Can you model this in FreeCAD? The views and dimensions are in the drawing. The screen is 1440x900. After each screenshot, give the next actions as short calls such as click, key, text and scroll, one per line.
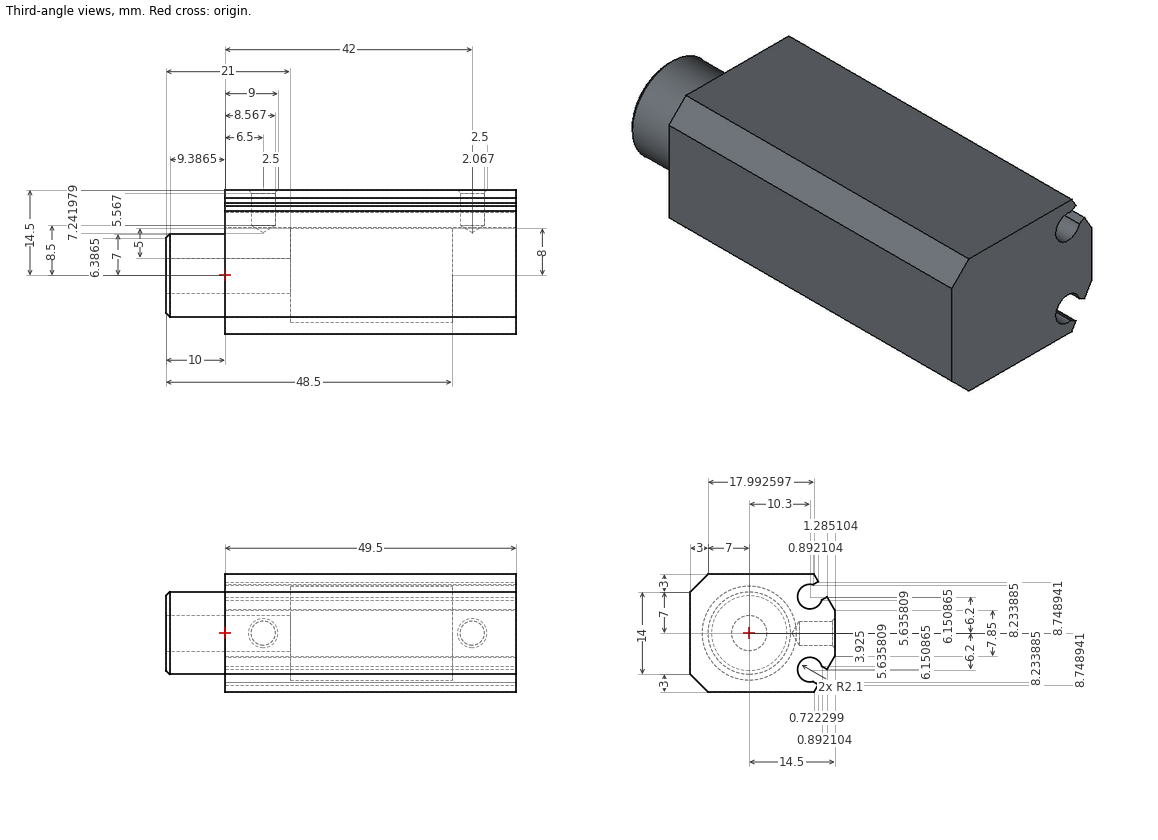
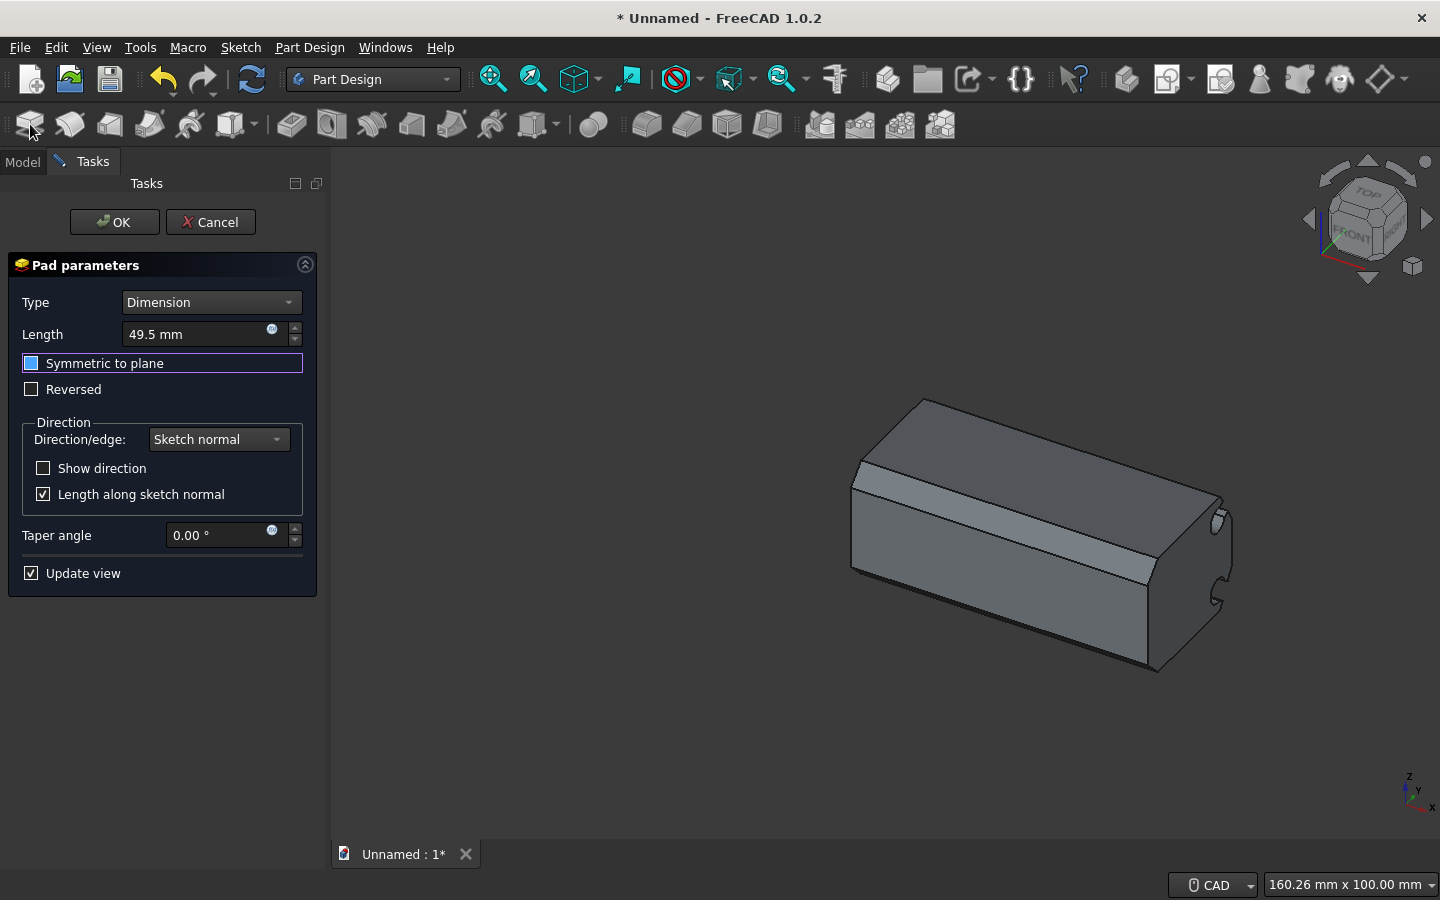
click(115, 222)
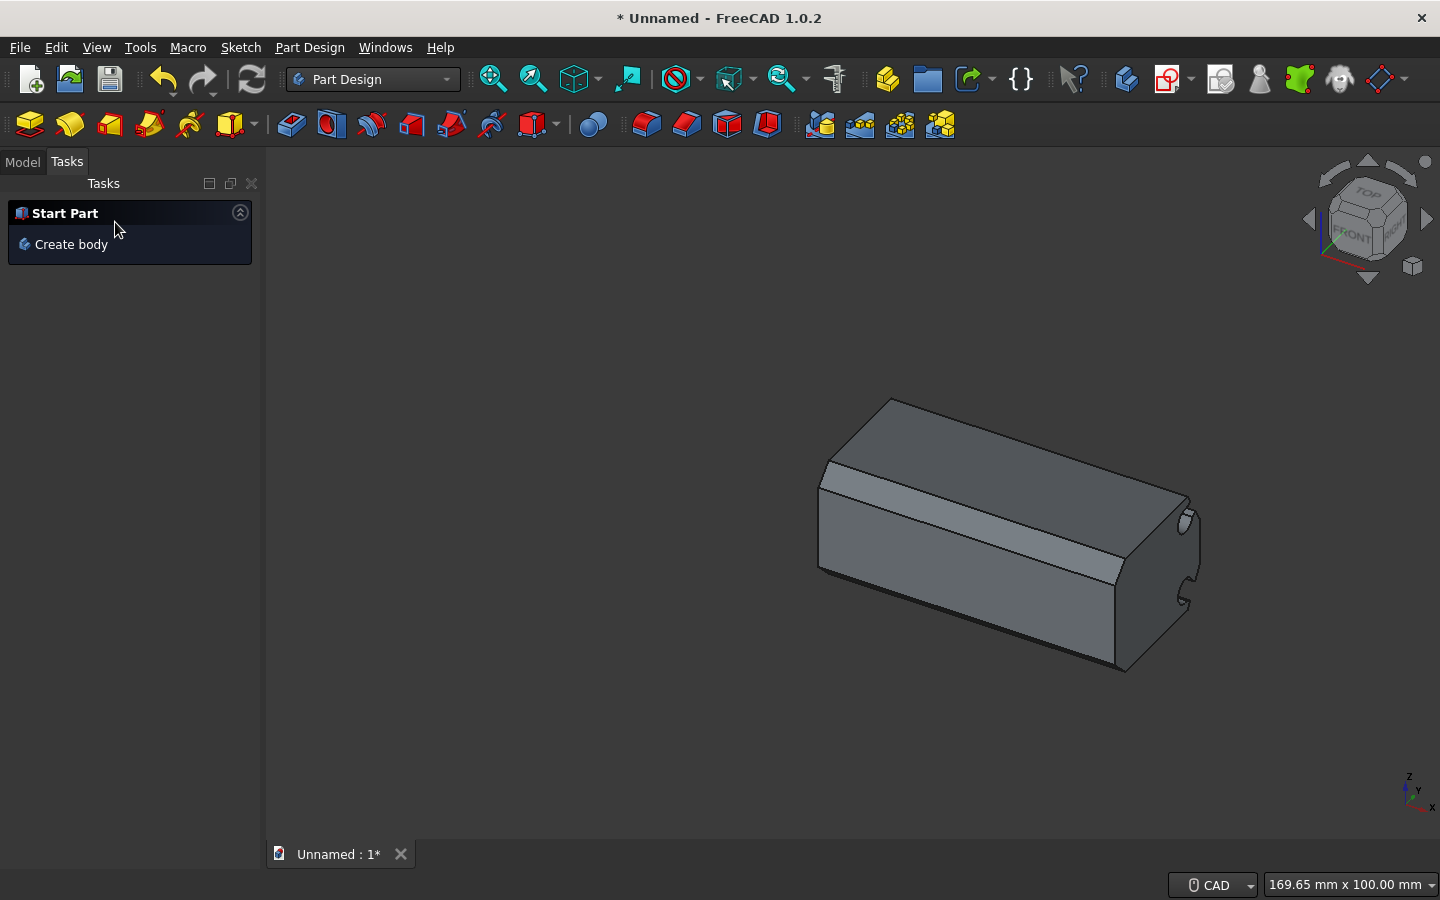
key(v)
key(f)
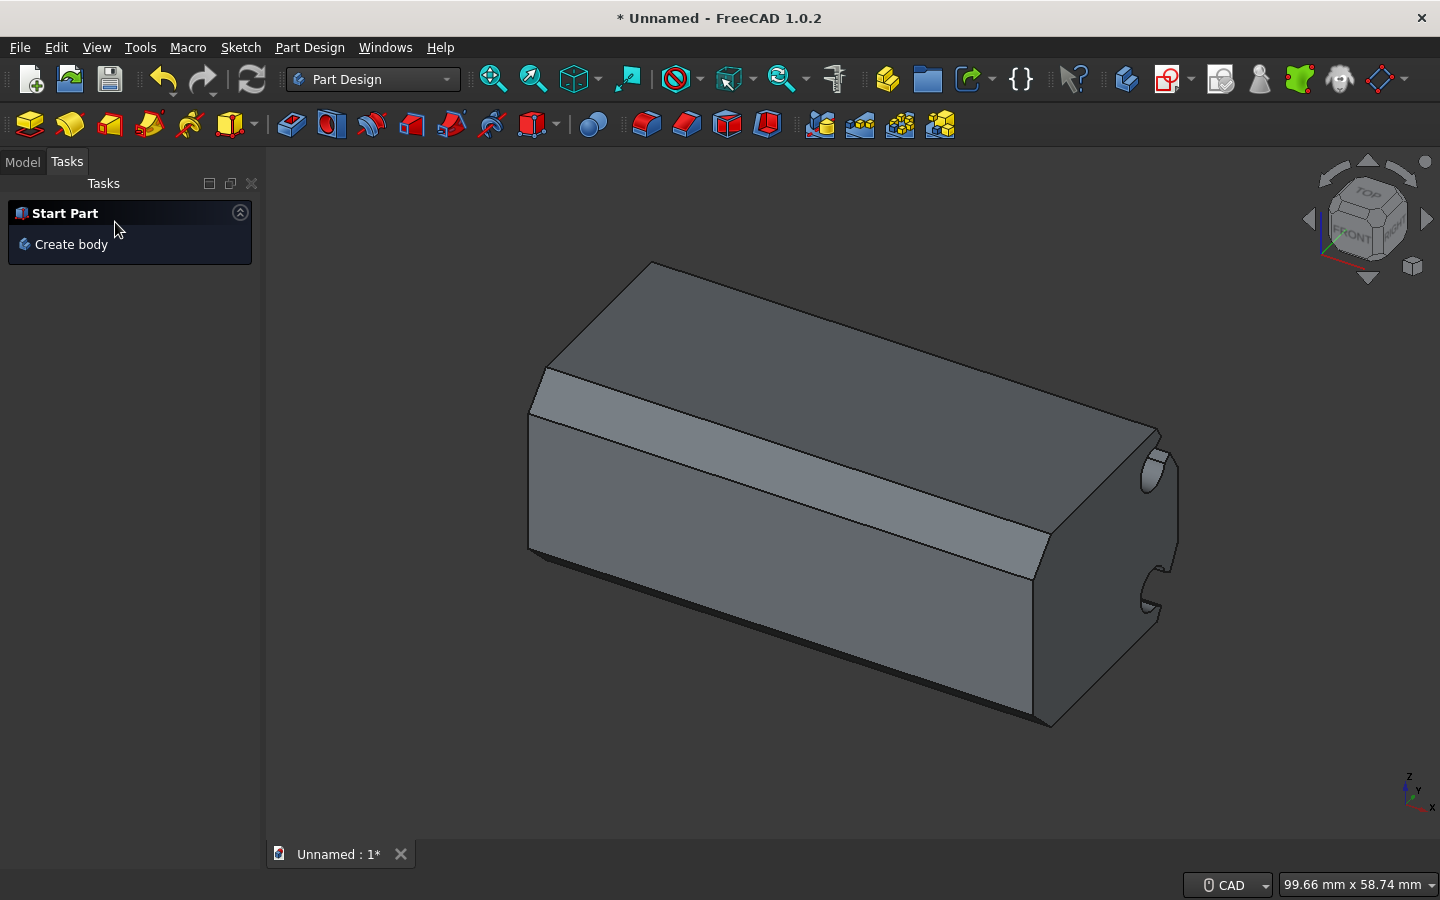
click(1168, 80)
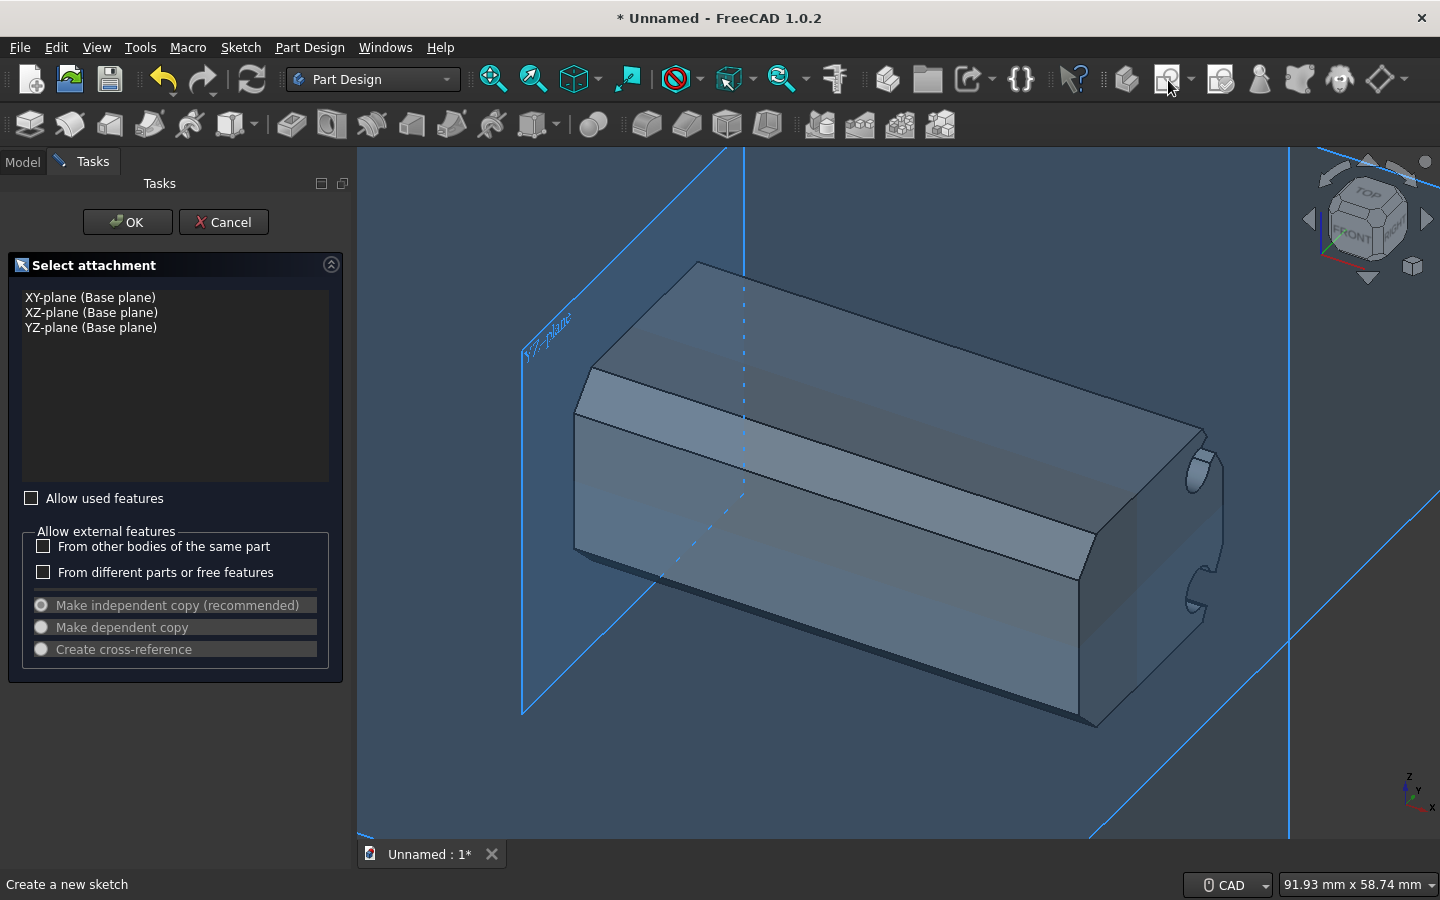
click(82, 298)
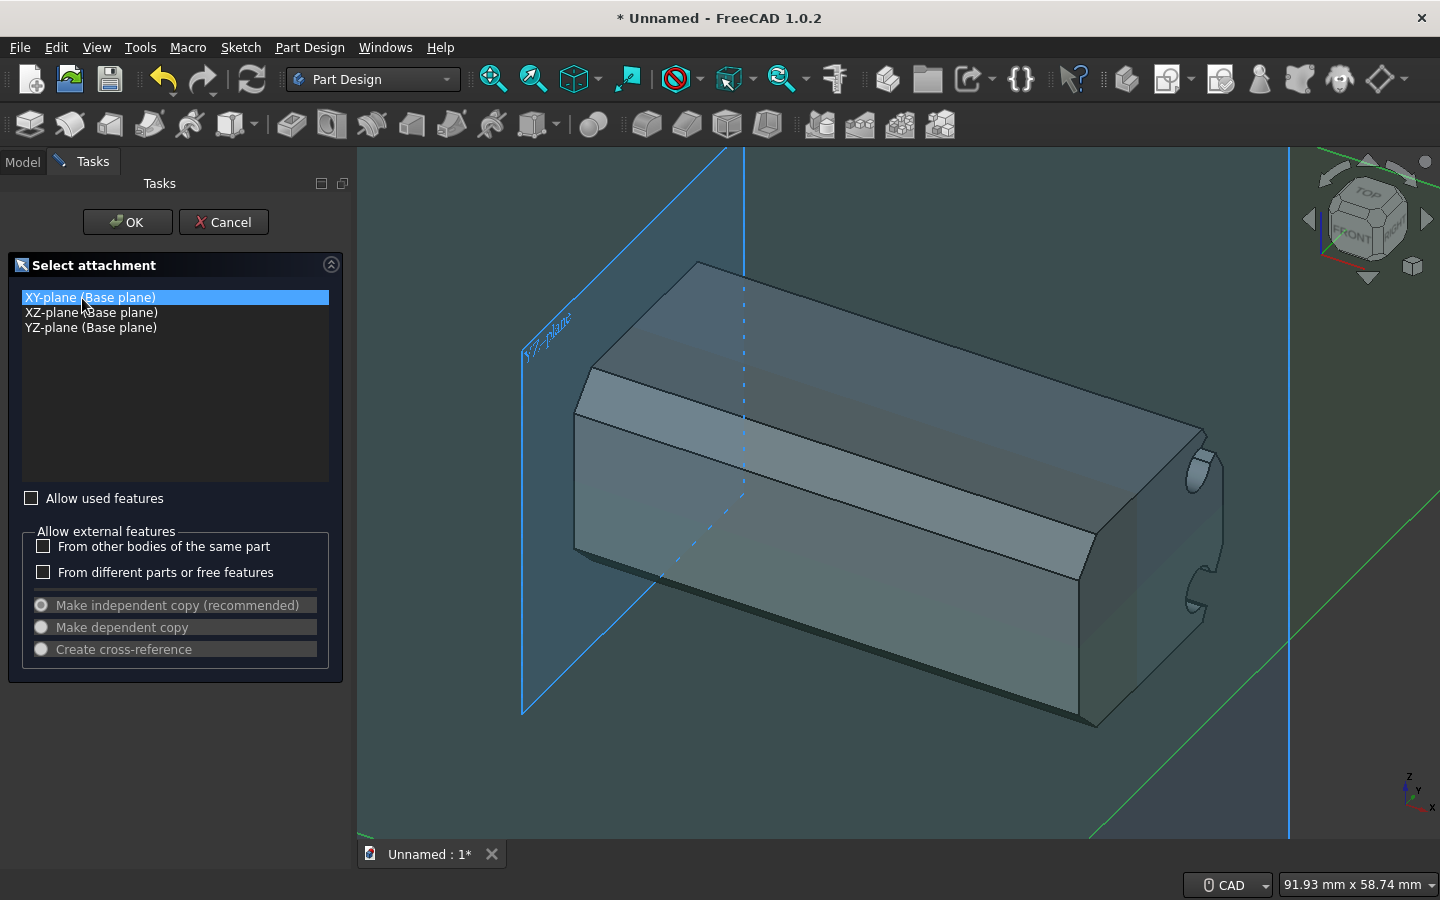
click(128, 222)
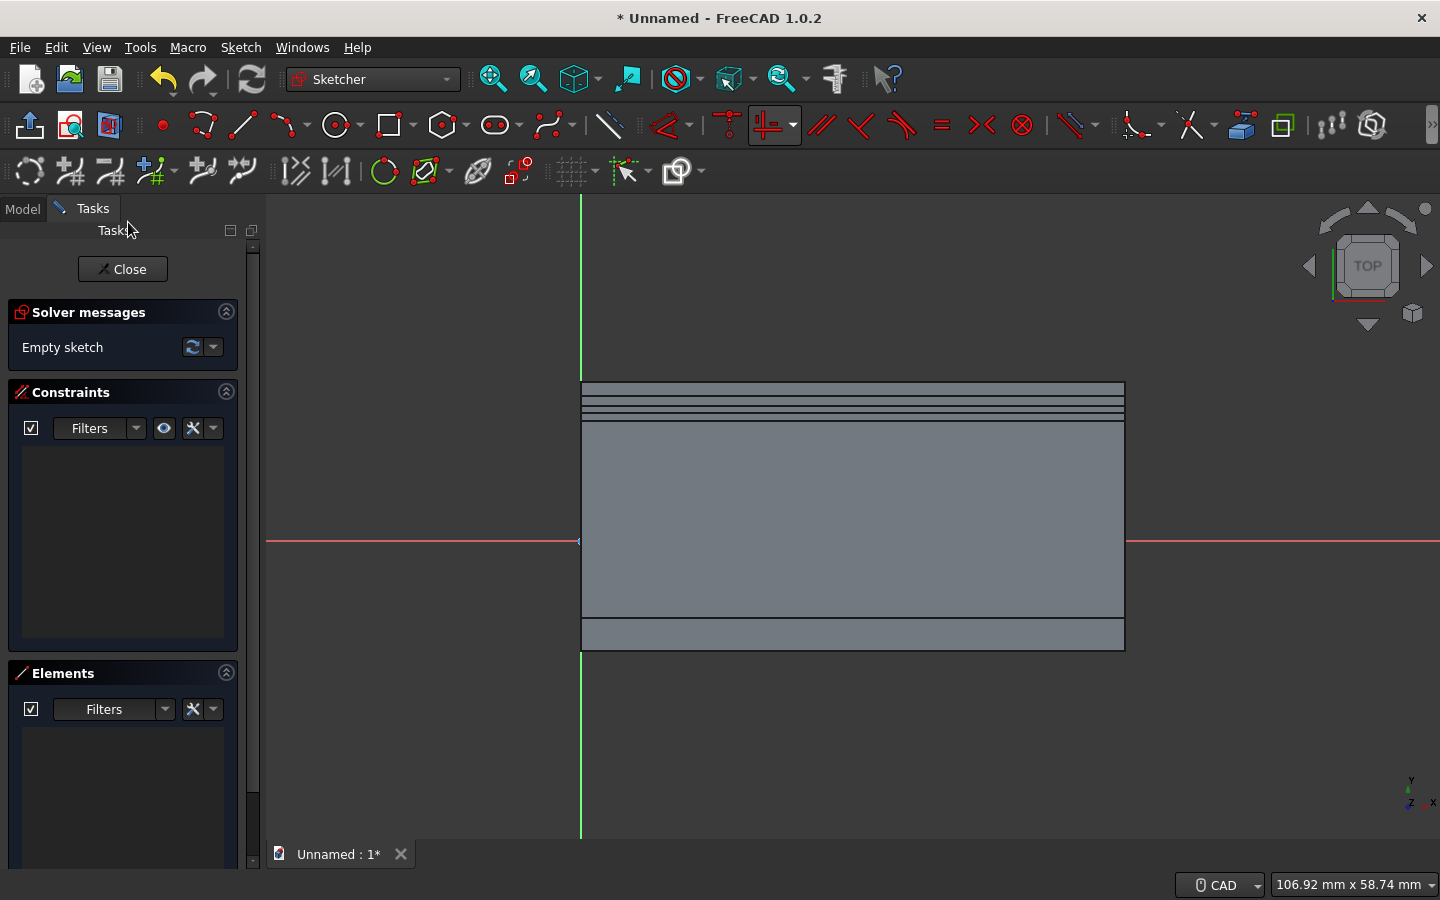
click(110, 126)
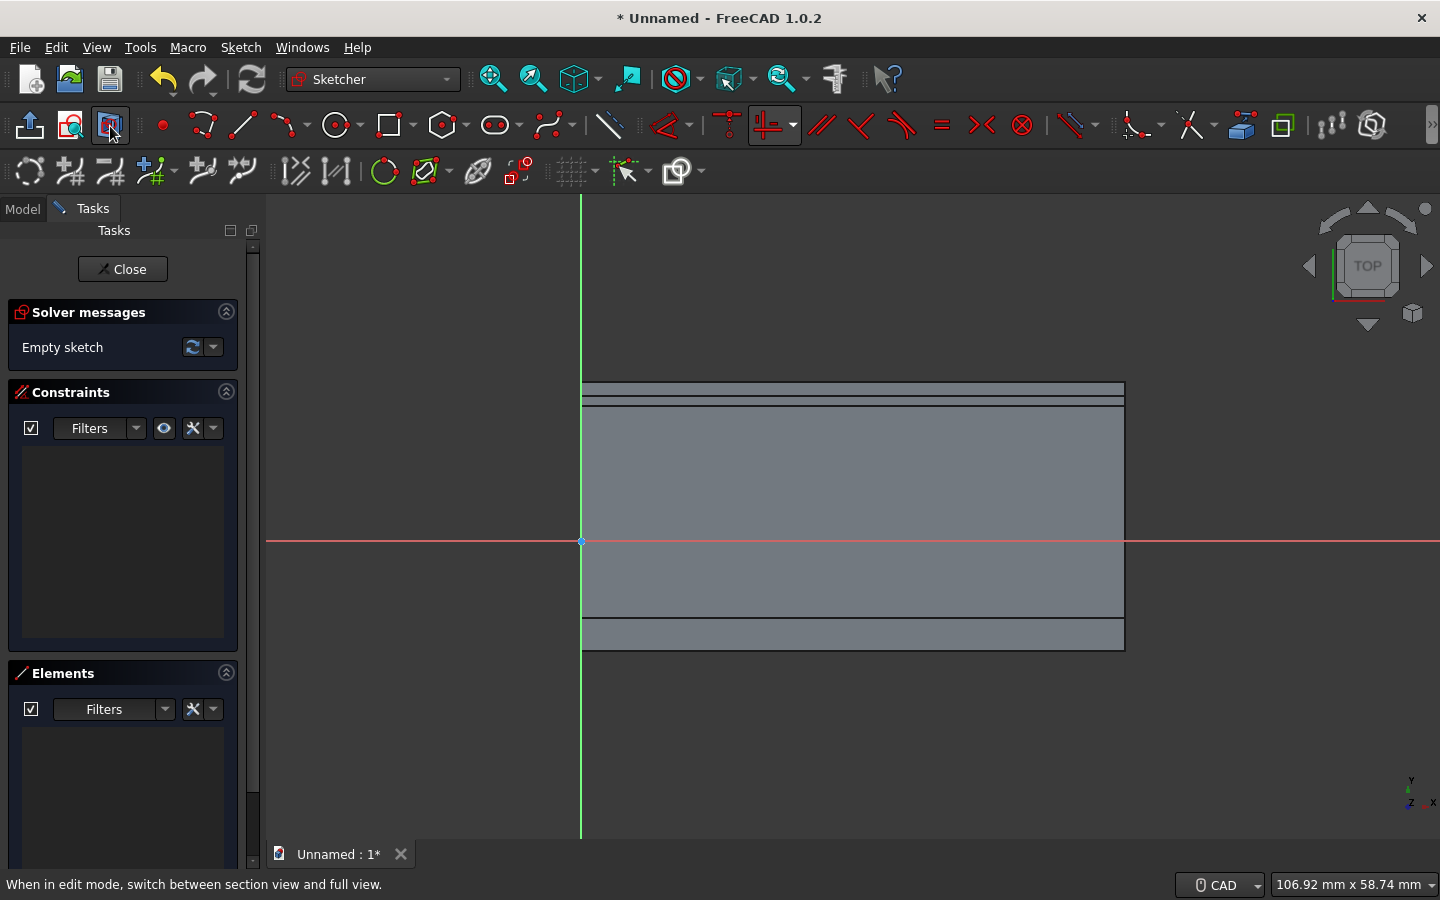
scroll(461, 499, up, 8)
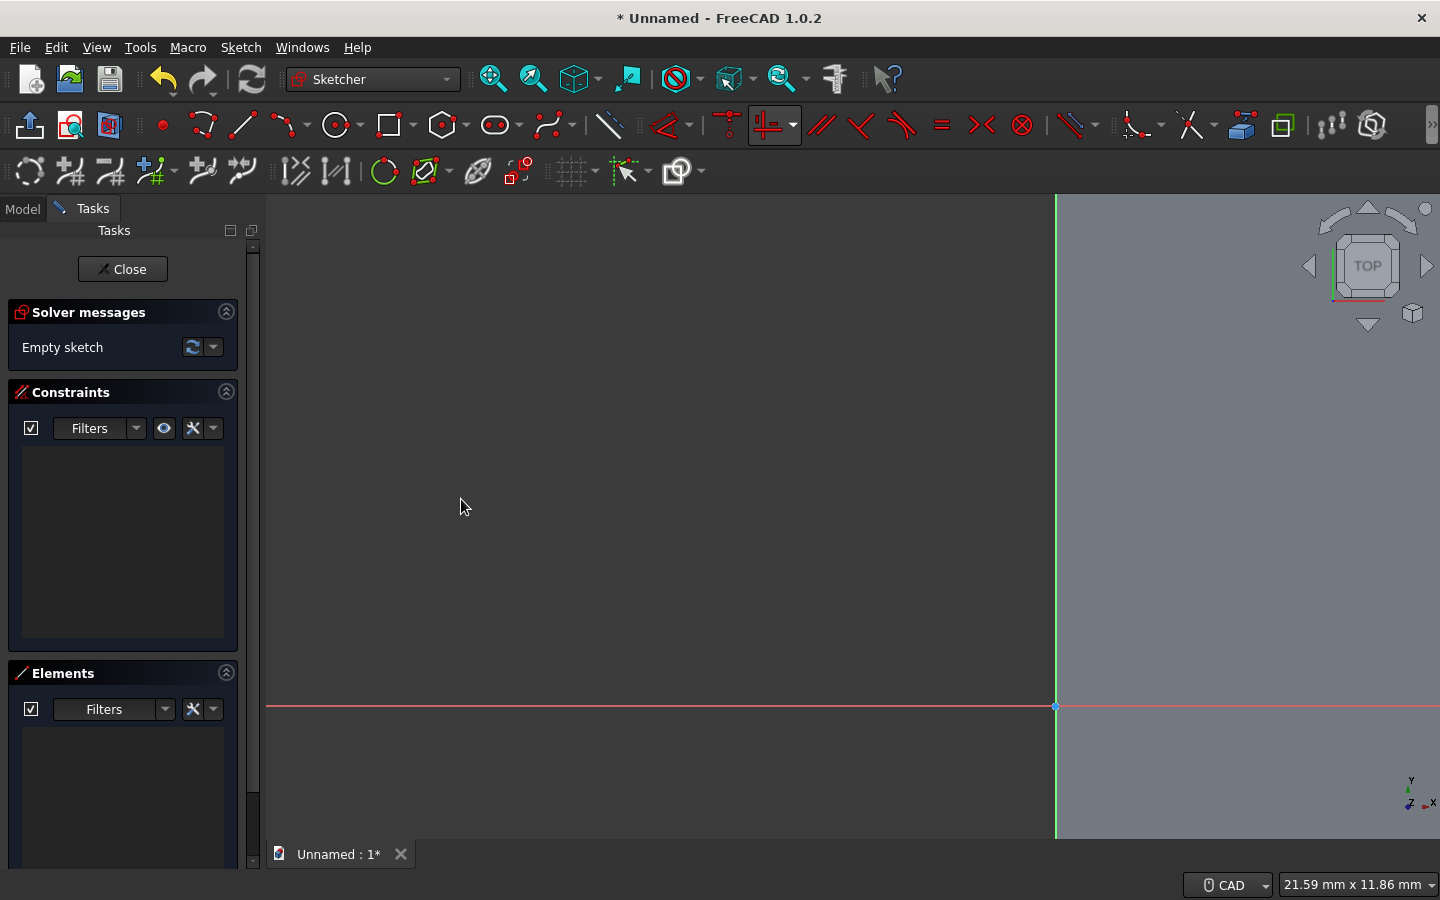
key(g)
key(m)